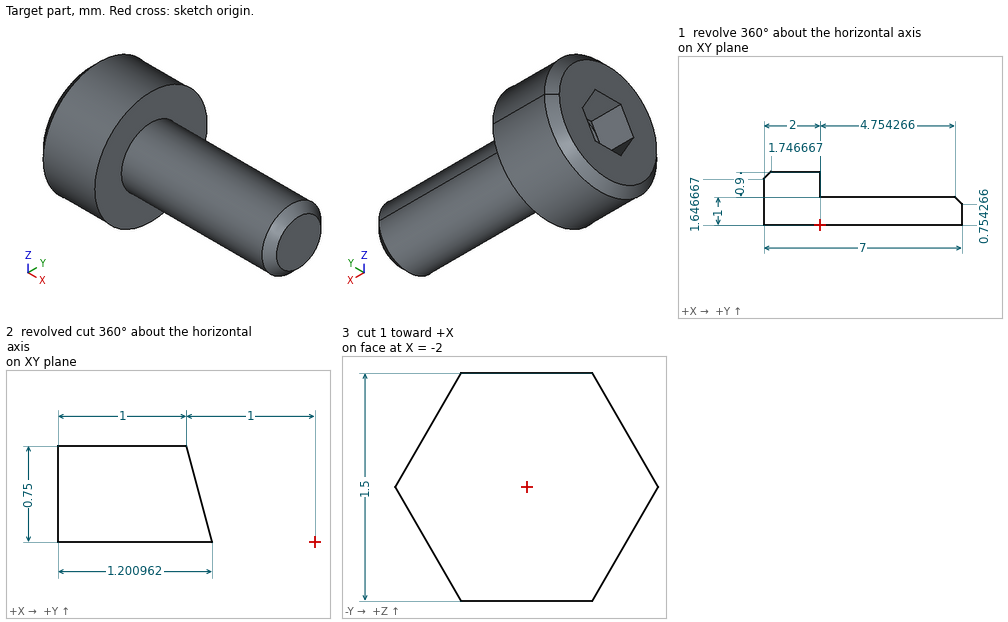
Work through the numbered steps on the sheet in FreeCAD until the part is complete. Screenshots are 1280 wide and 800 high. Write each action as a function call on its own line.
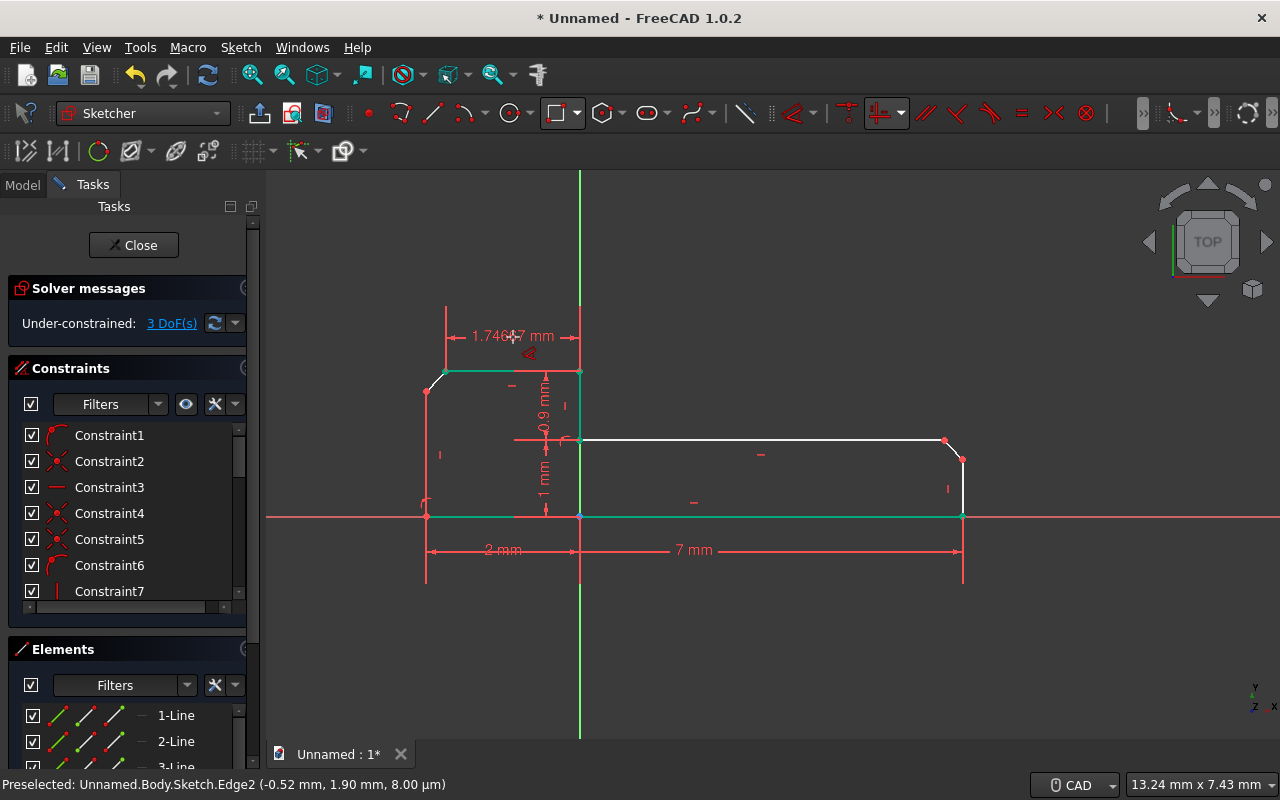
click(426, 429)
click(392, 454)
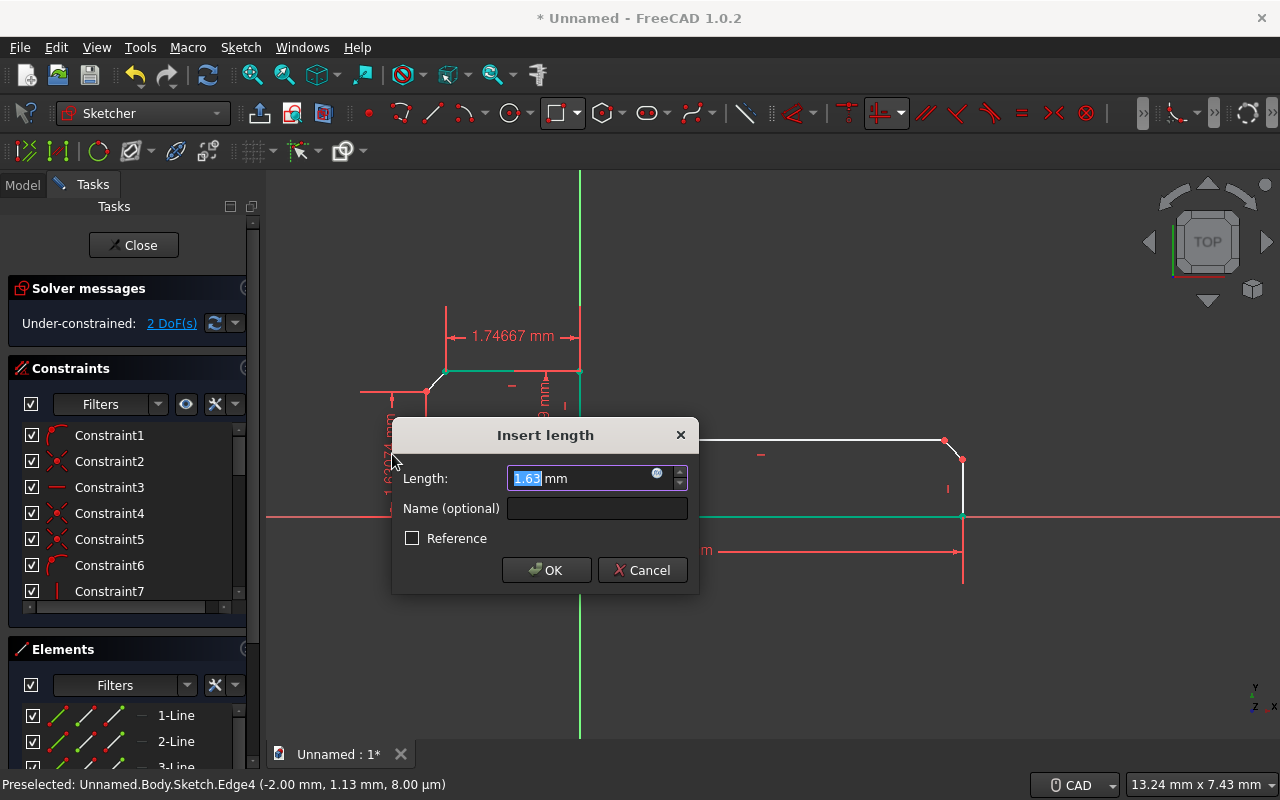
text(1.646667)
key(Return)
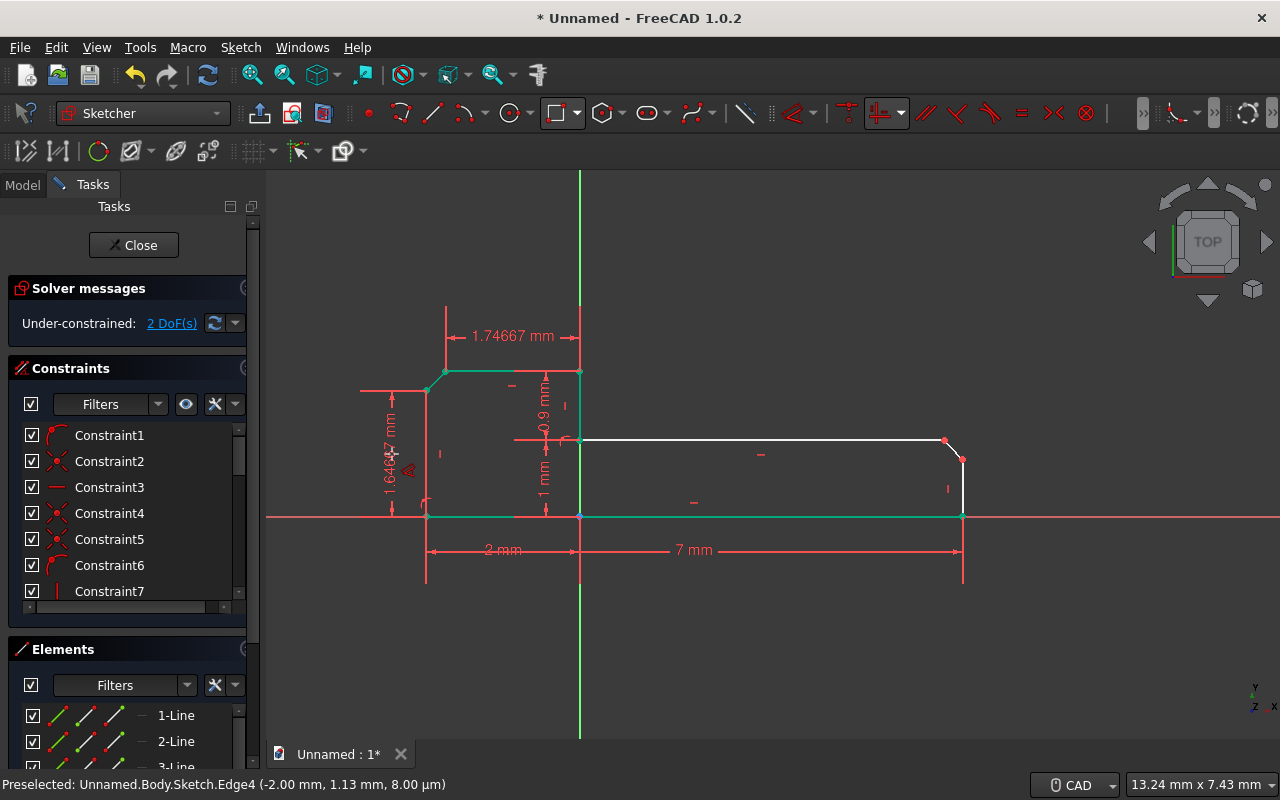
click(963, 500)
click(997, 488)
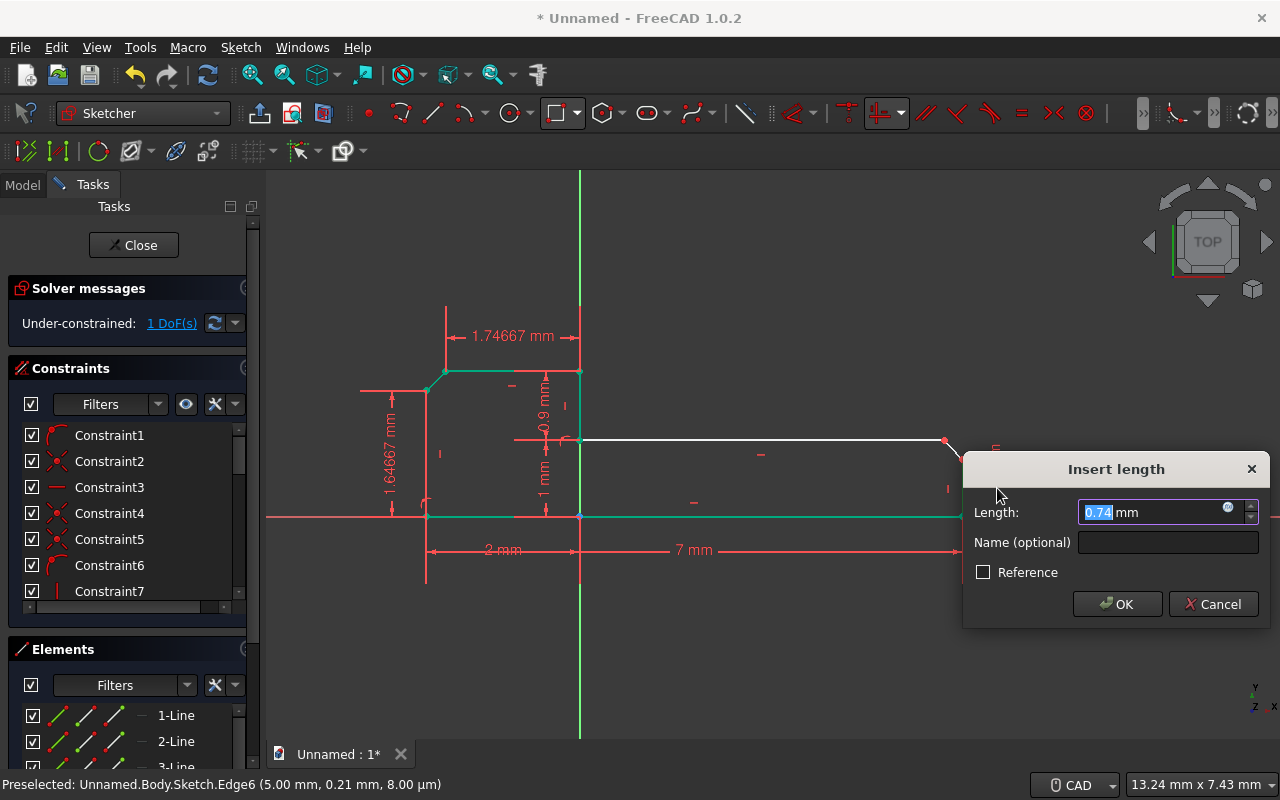
text(0.754266)
key(Return)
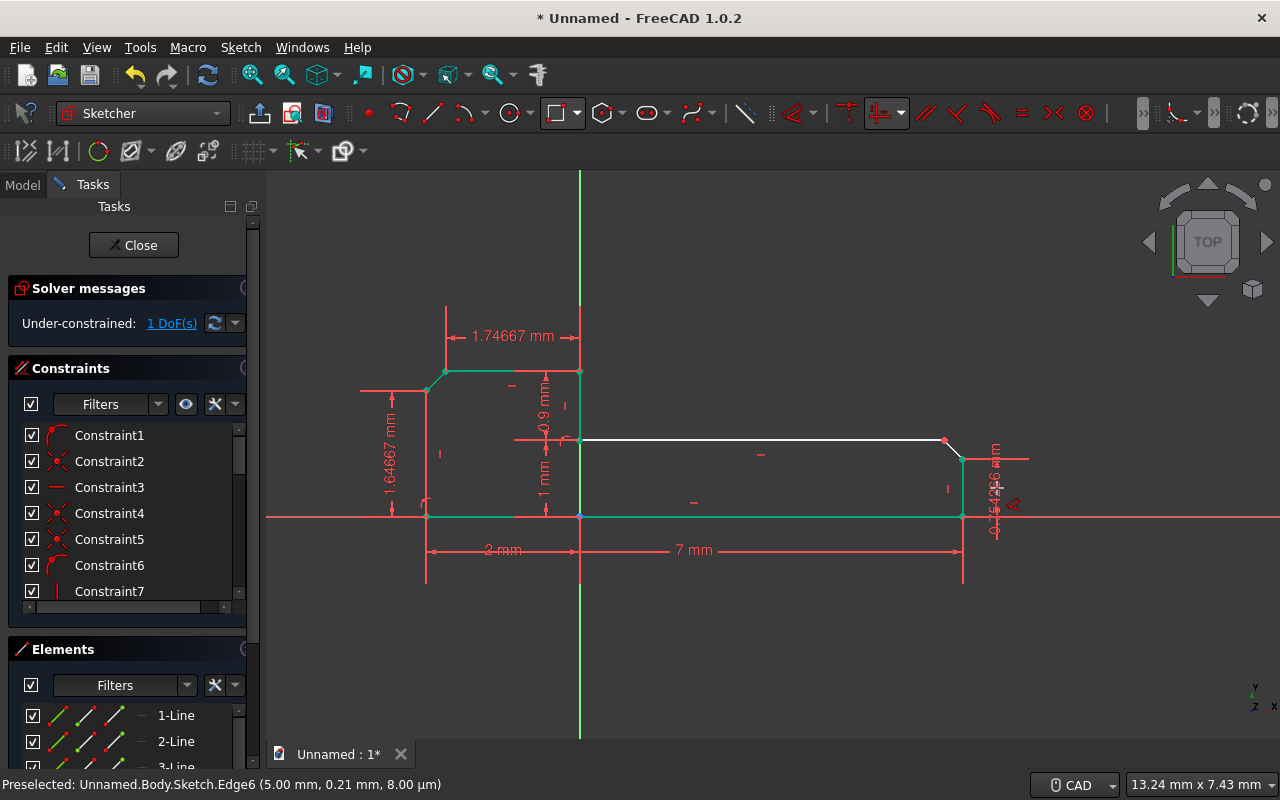
click(835, 440)
click(762, 406)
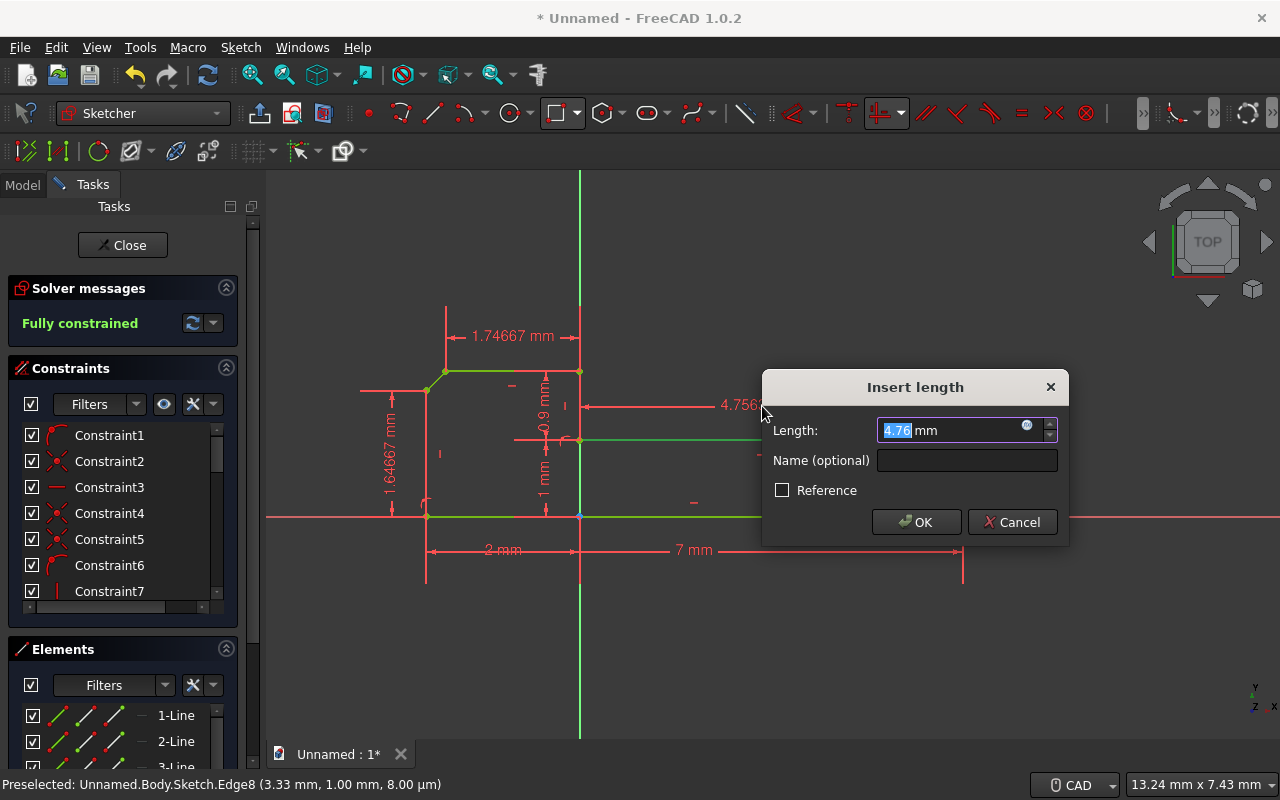
text(4.754266)
key(Return)
key(Escape)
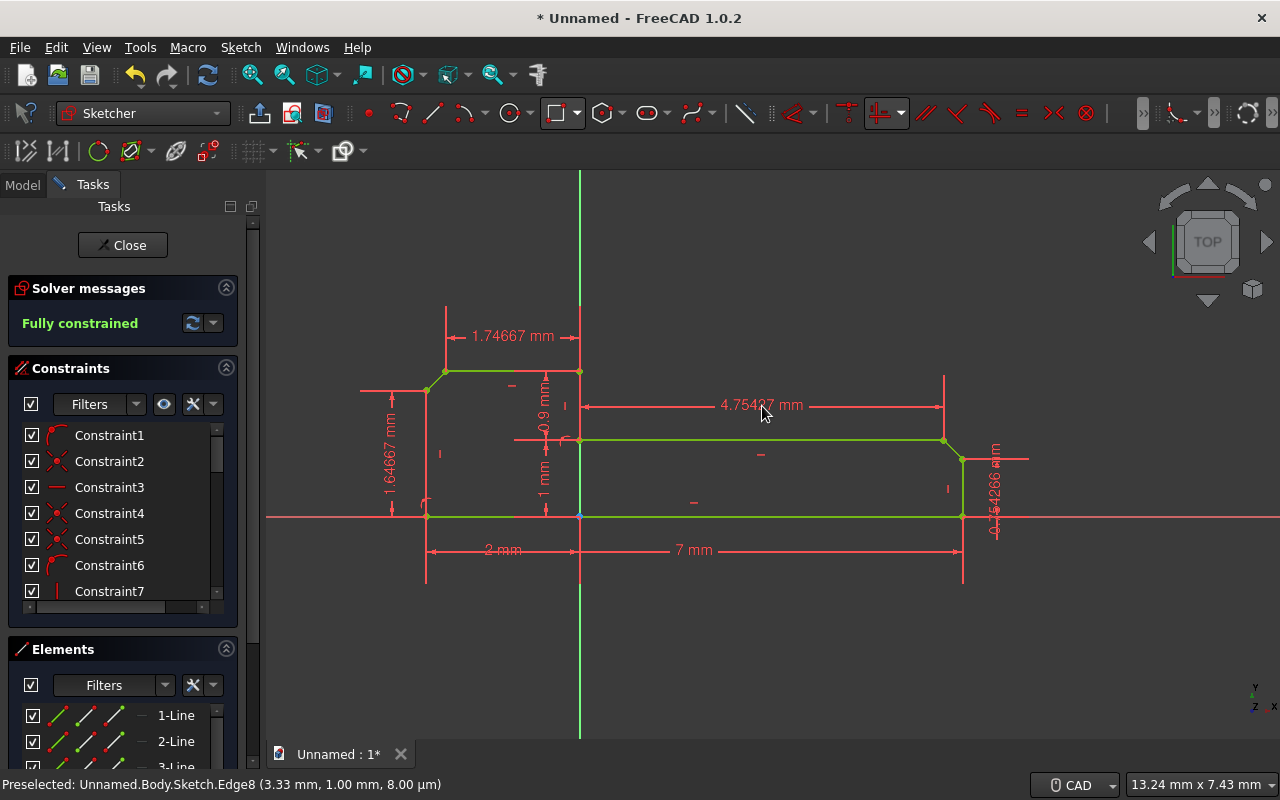
click(123, 245)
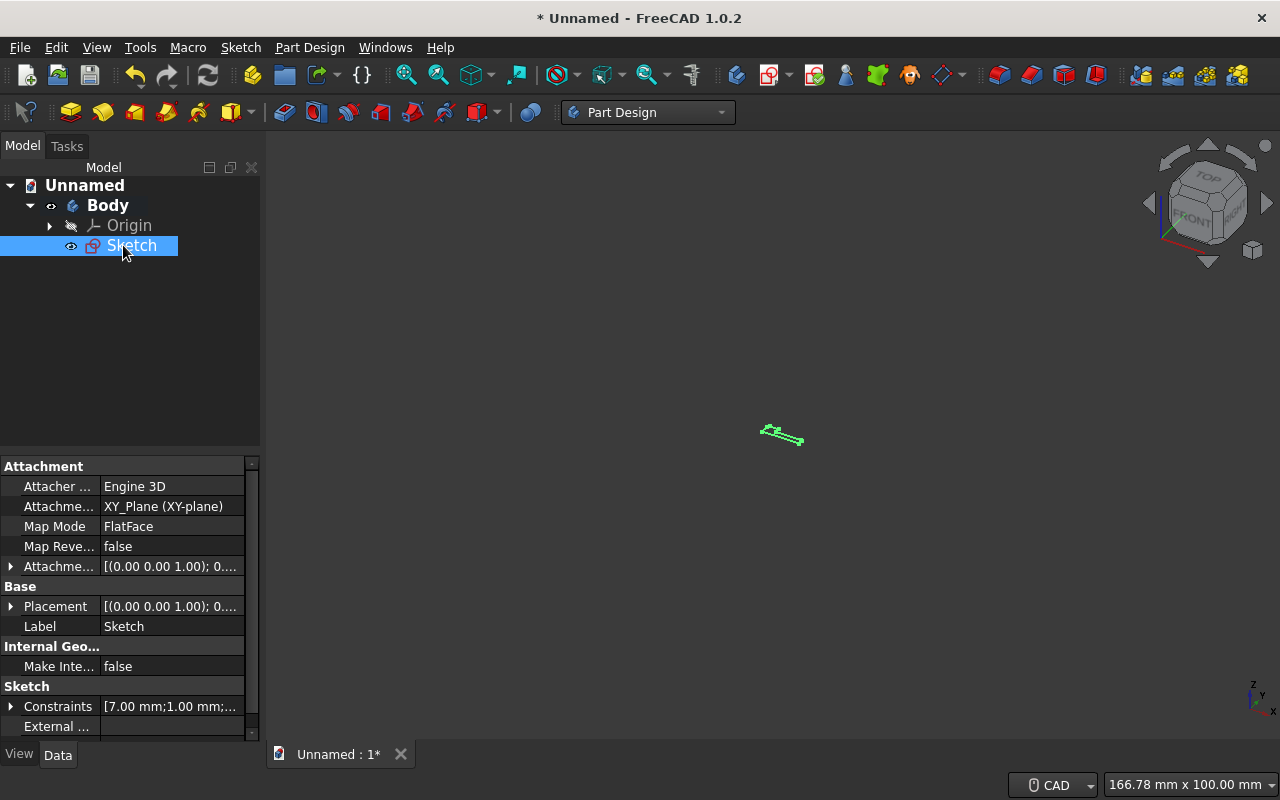
click(104, 112)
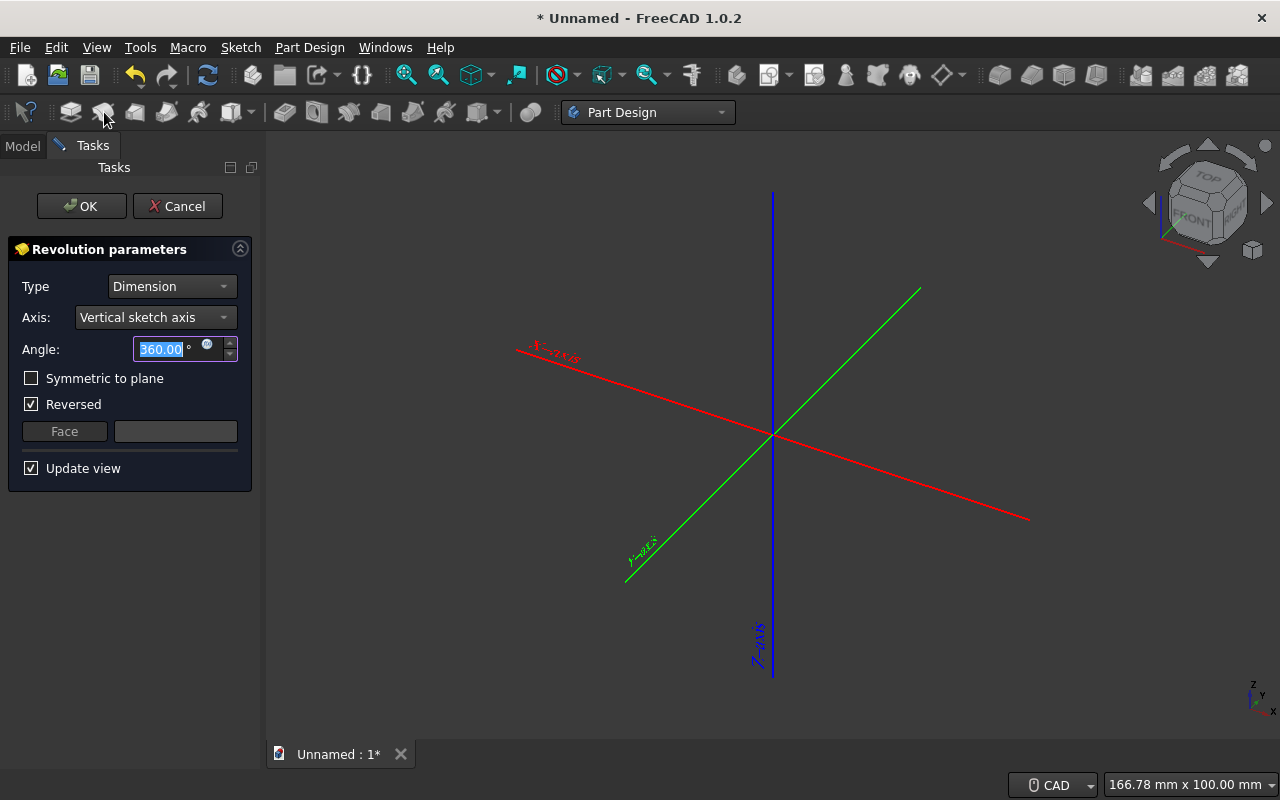
click(156, 318)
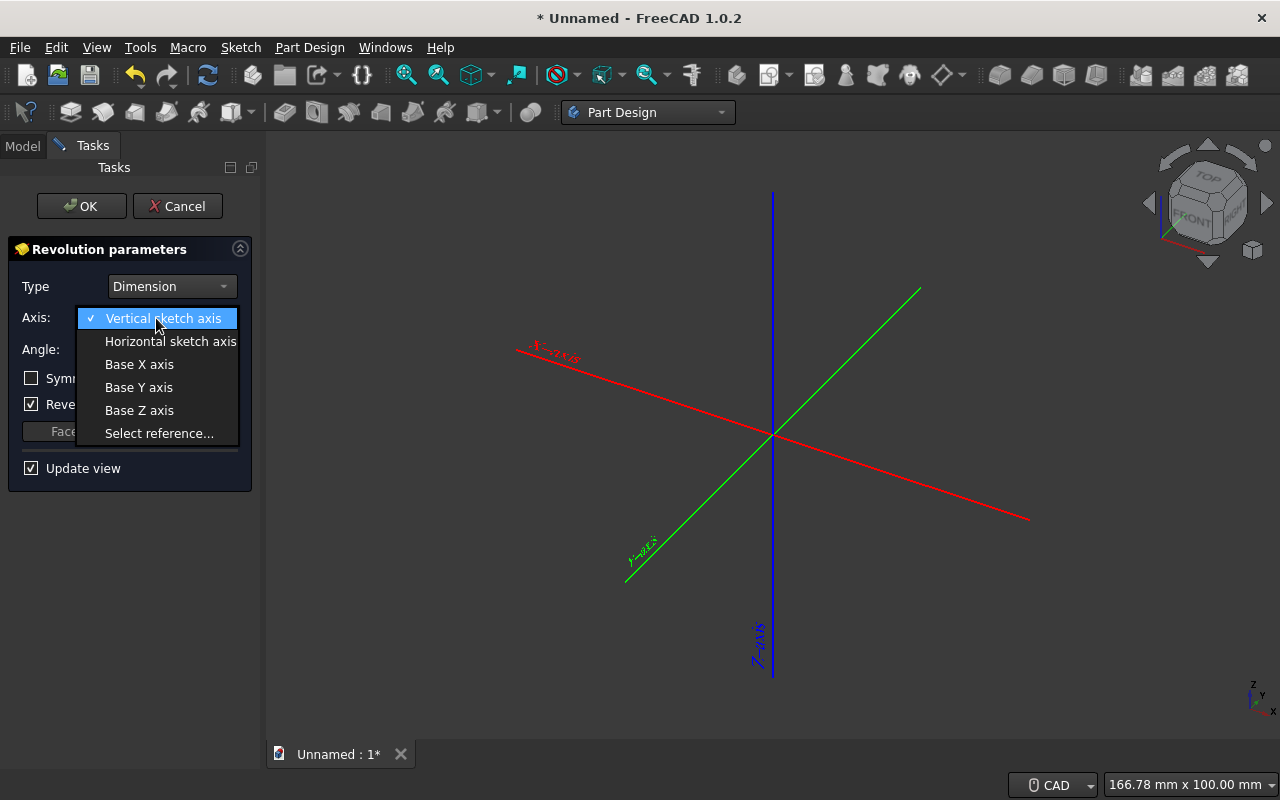
click(156, 342)